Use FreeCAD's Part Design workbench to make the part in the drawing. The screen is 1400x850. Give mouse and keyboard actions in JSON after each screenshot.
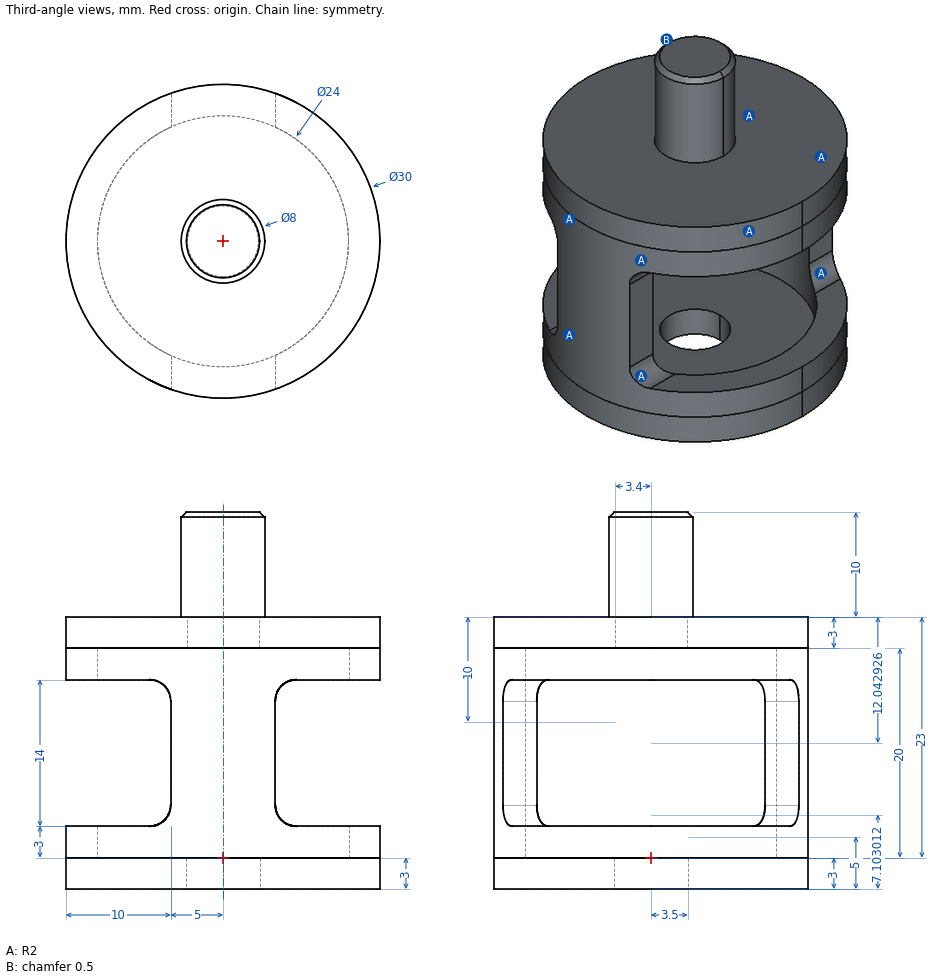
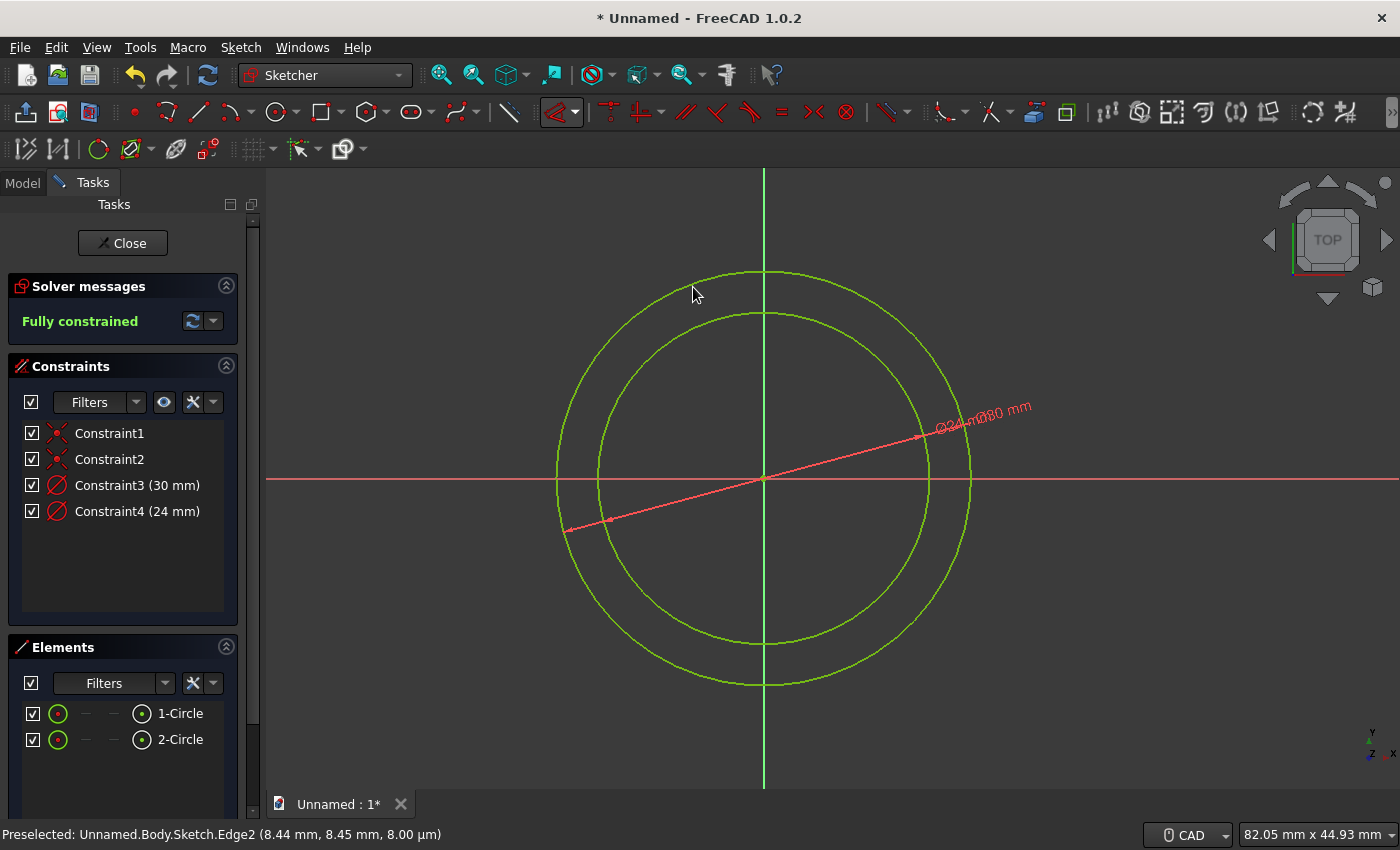
{"action": "left_click", "coordinate": [123, 243]}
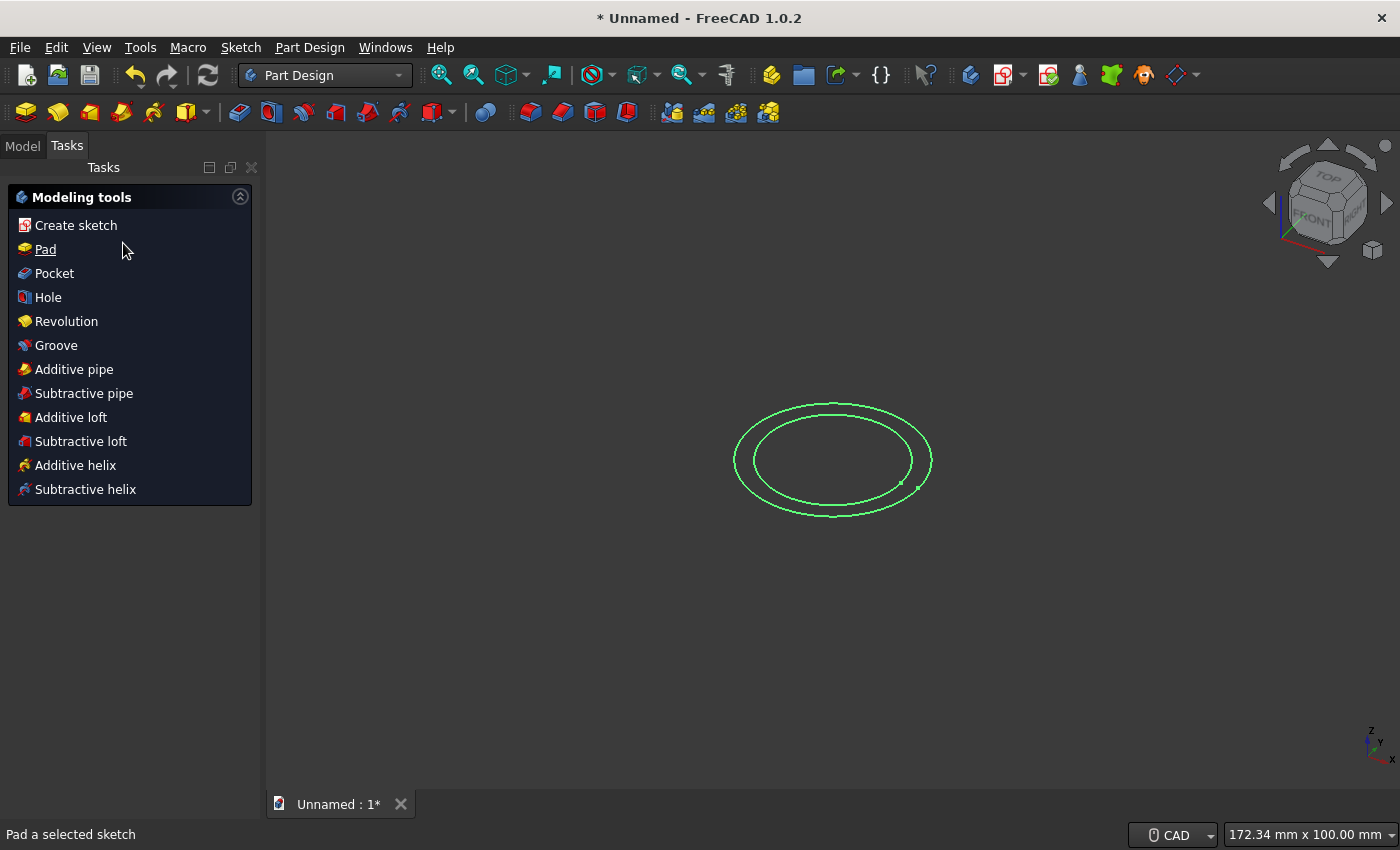
{"action": "left_click", "coordinate": [26, 112]}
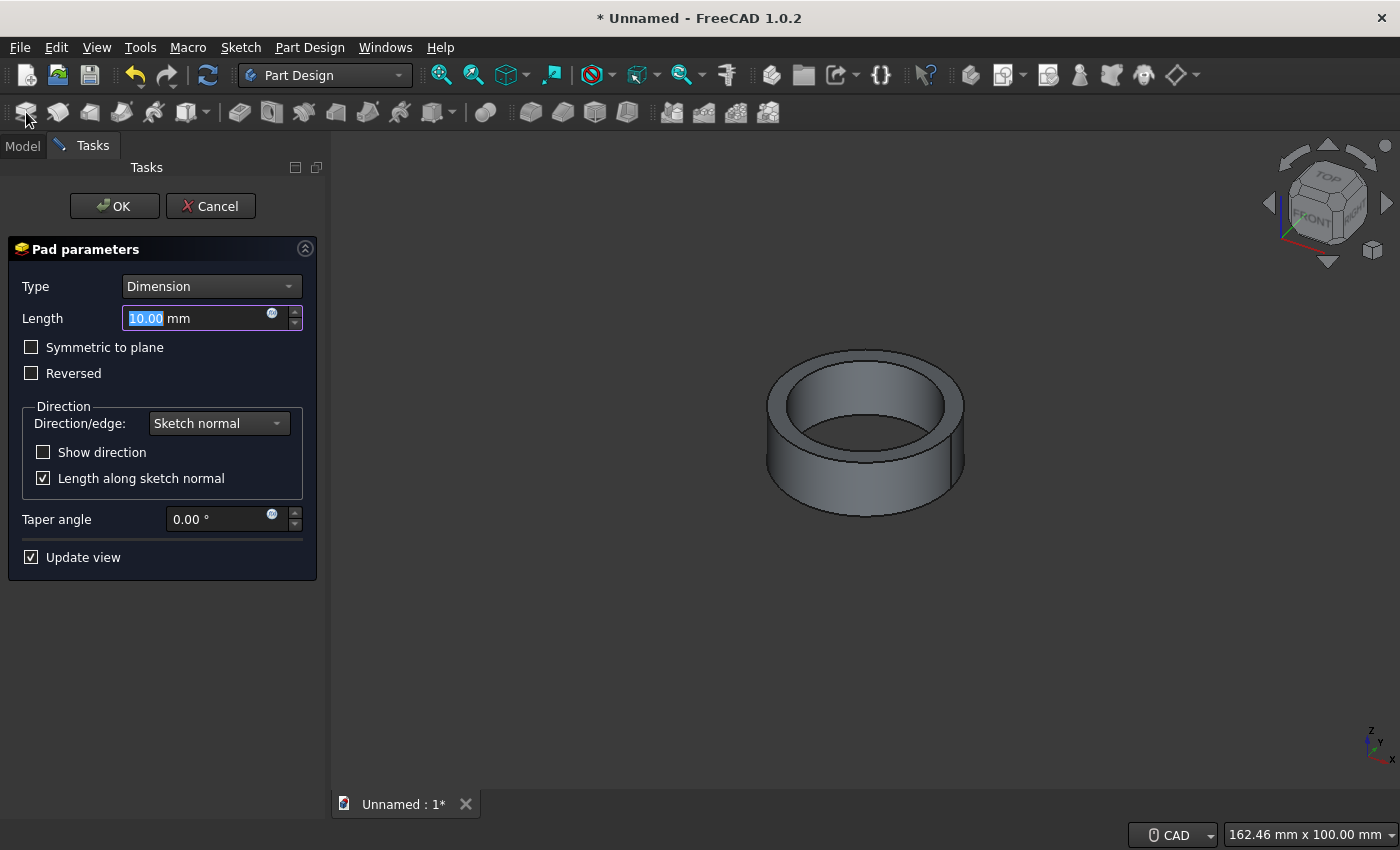
{"action": "type", "text": "20"}
{"action": "key", "text": "Tab"}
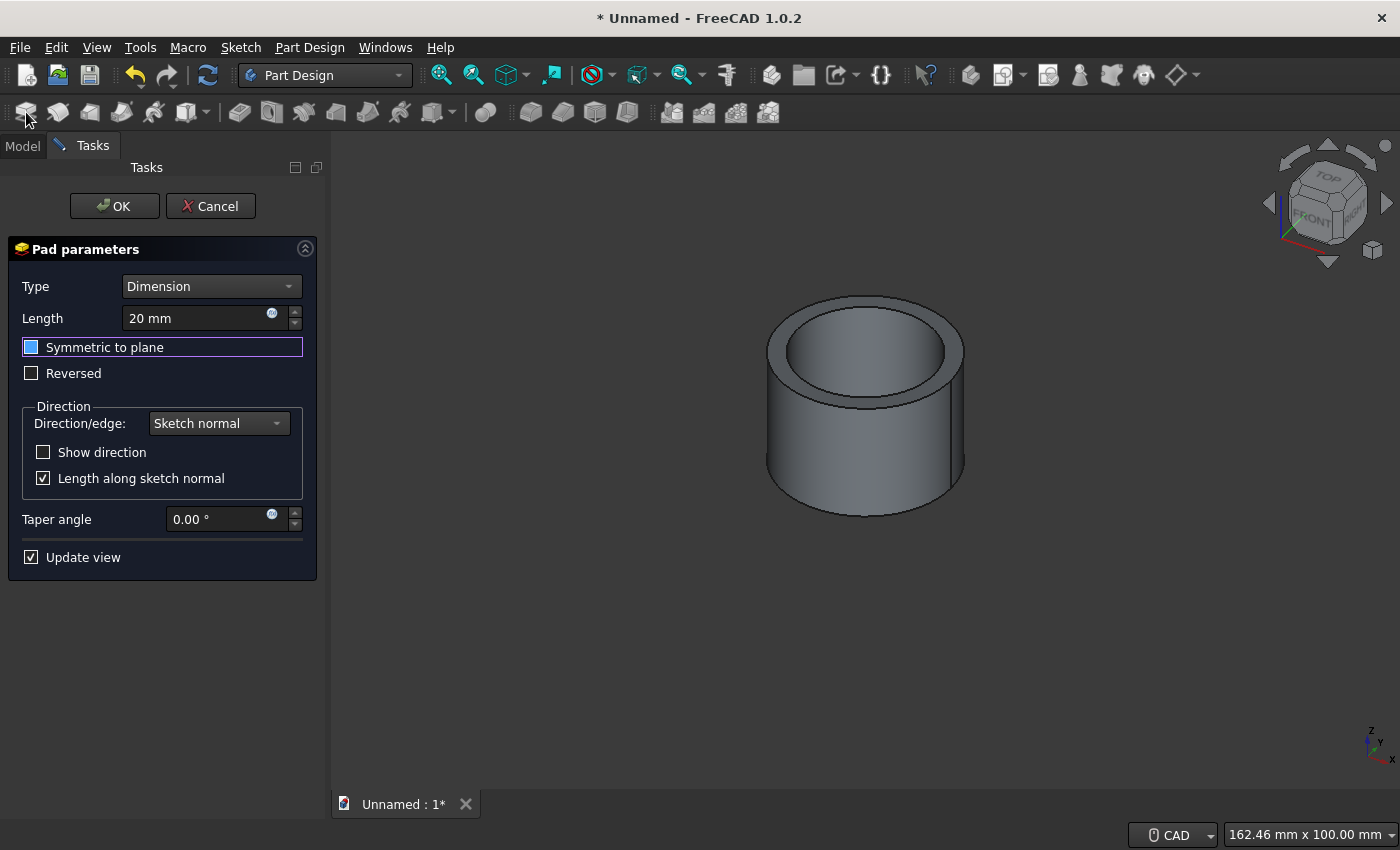
{"action": "left_click", "coordinate": [115, 206]}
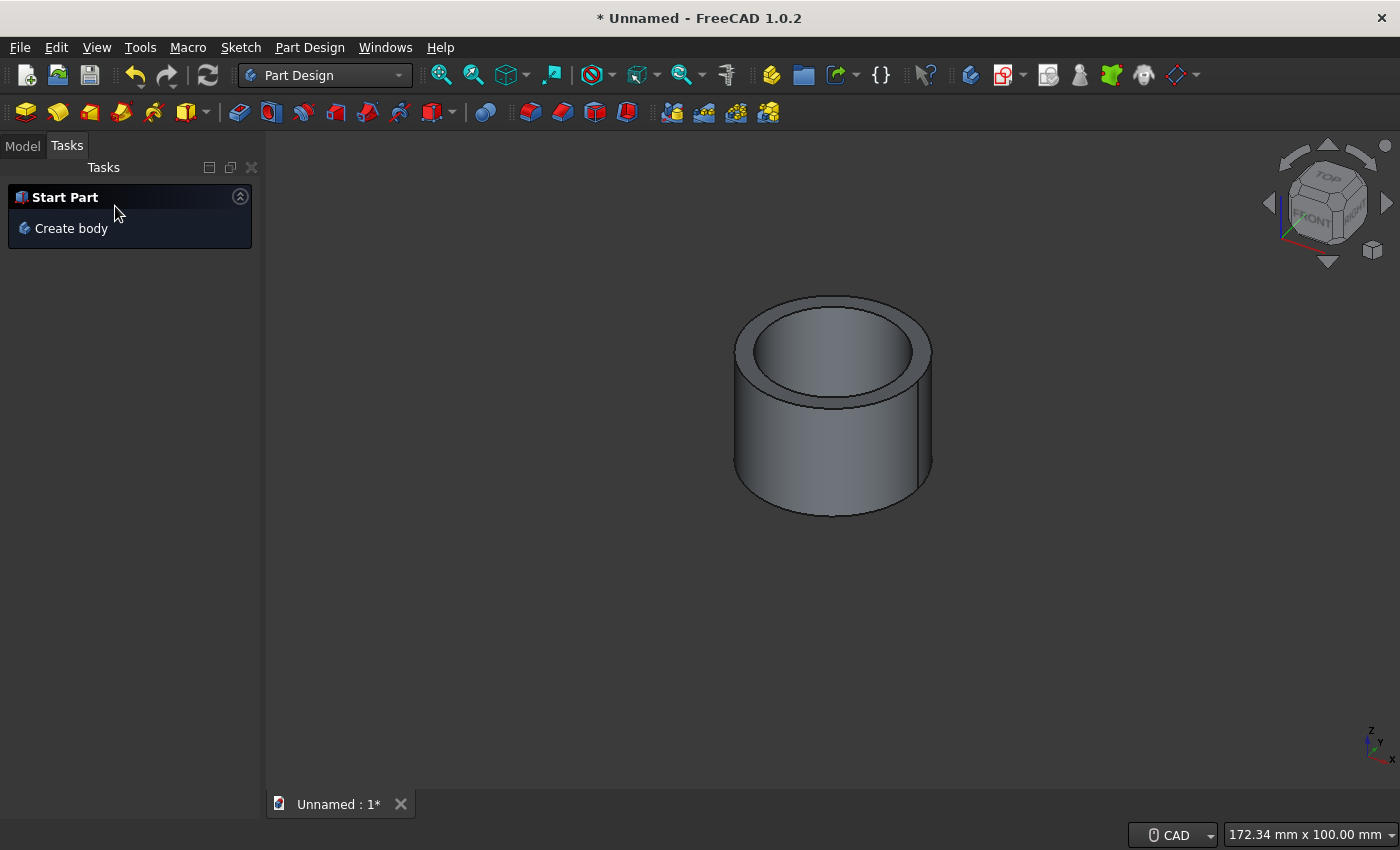
{"action": "left_click", "coordinate": [442, 76]}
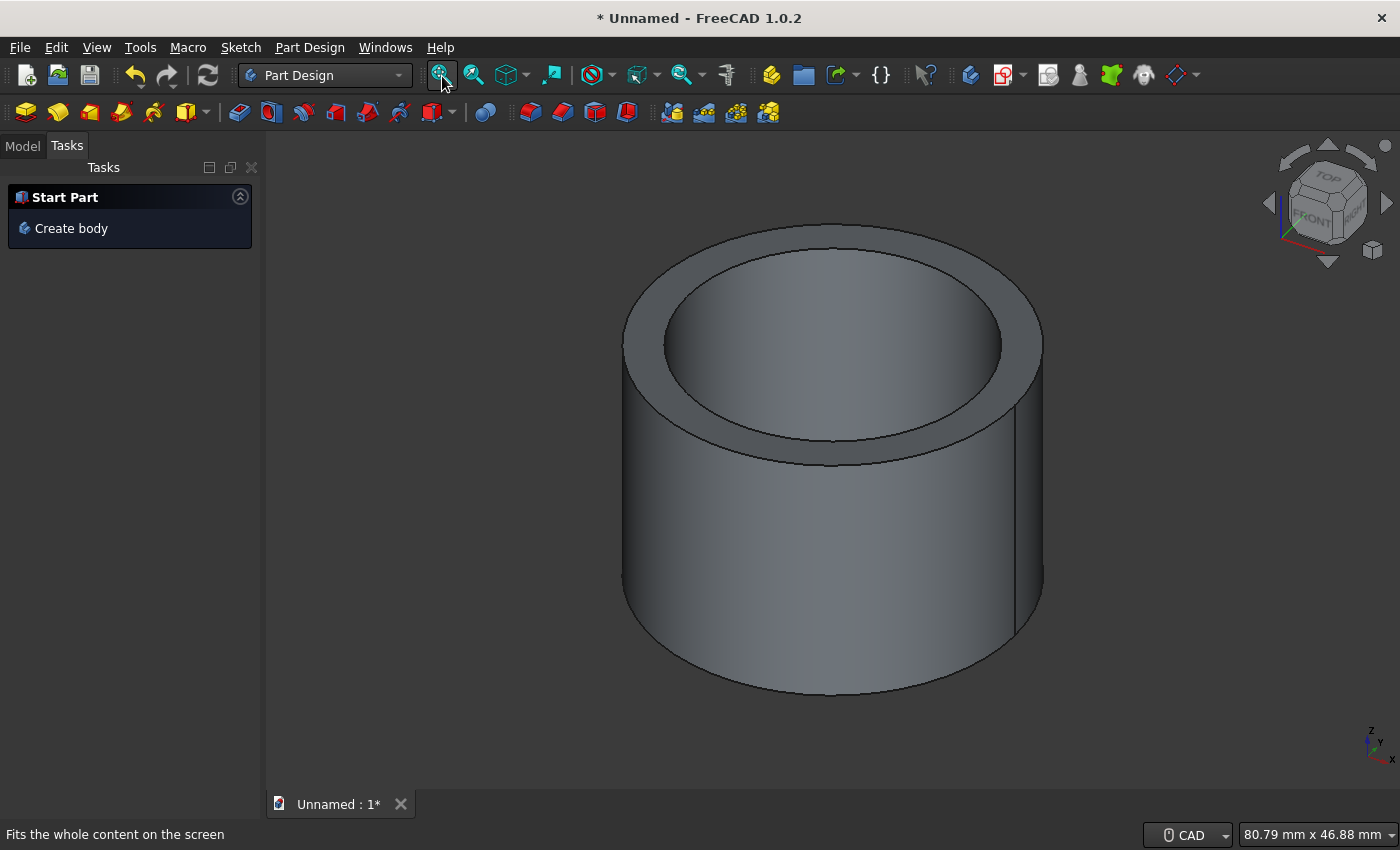
{"action": "left_click", "coordinate": [1004, 76]}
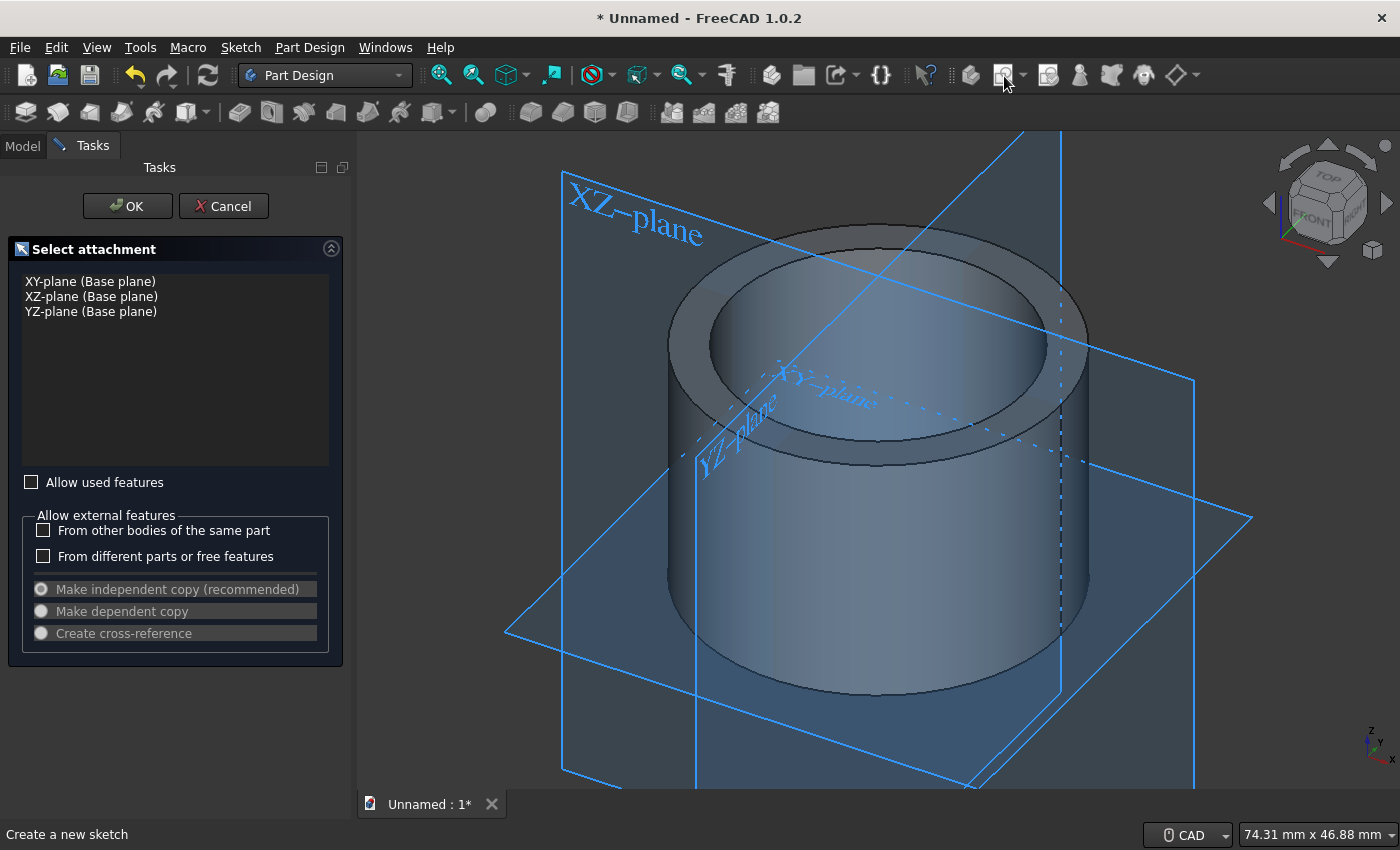
{"action": "left_click", "coordinate": [82, 296]}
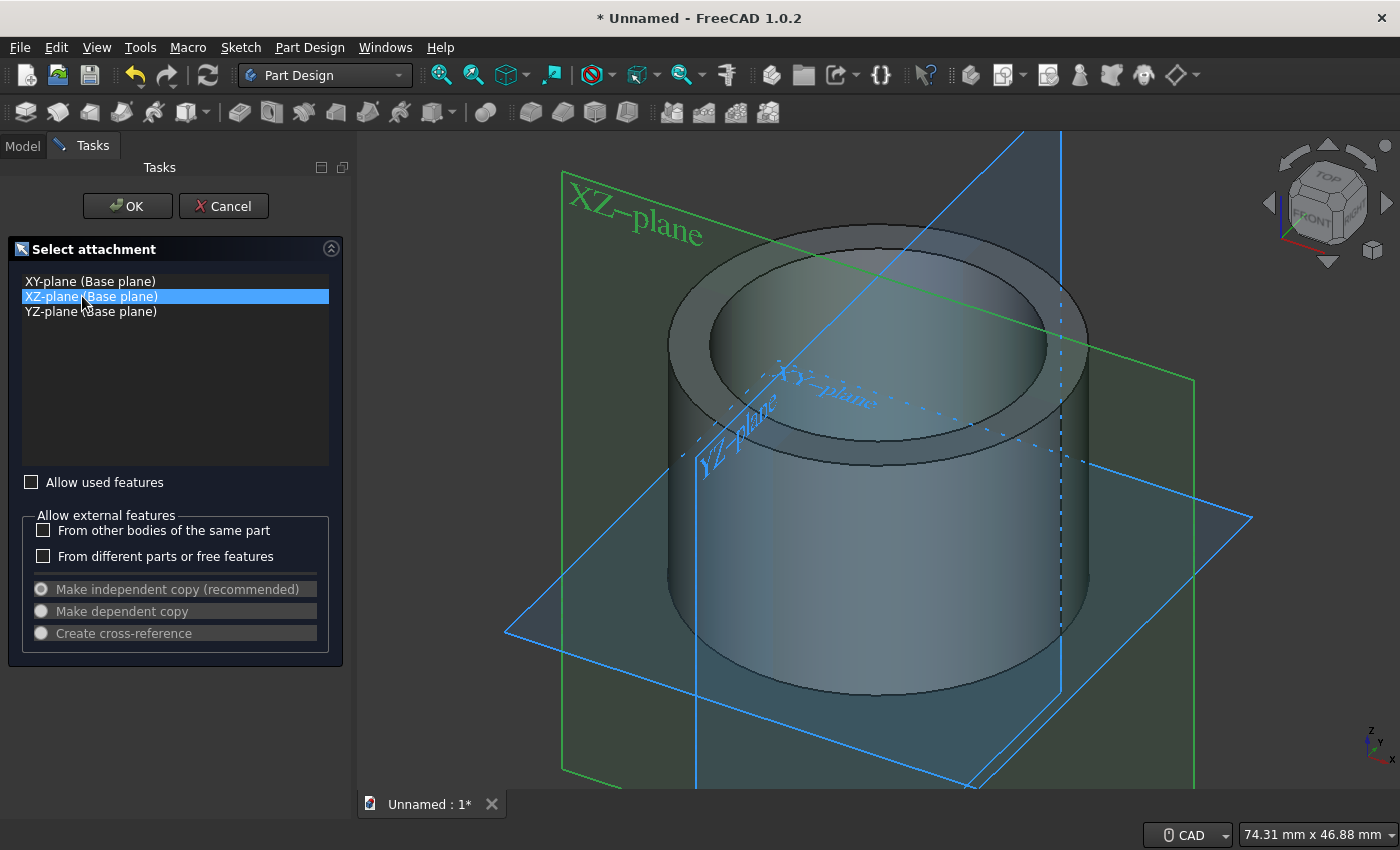
{"action": "left_click", "coordinate": [128, 206]}